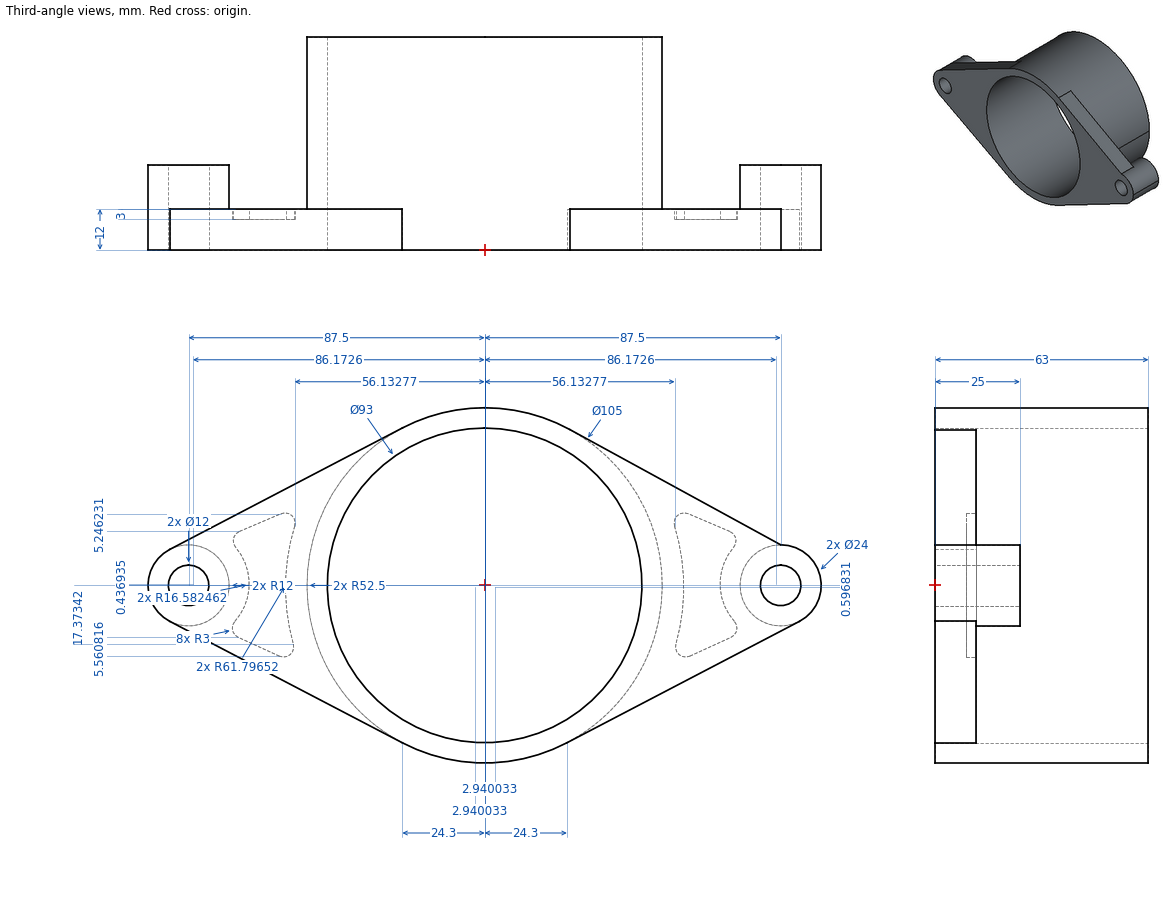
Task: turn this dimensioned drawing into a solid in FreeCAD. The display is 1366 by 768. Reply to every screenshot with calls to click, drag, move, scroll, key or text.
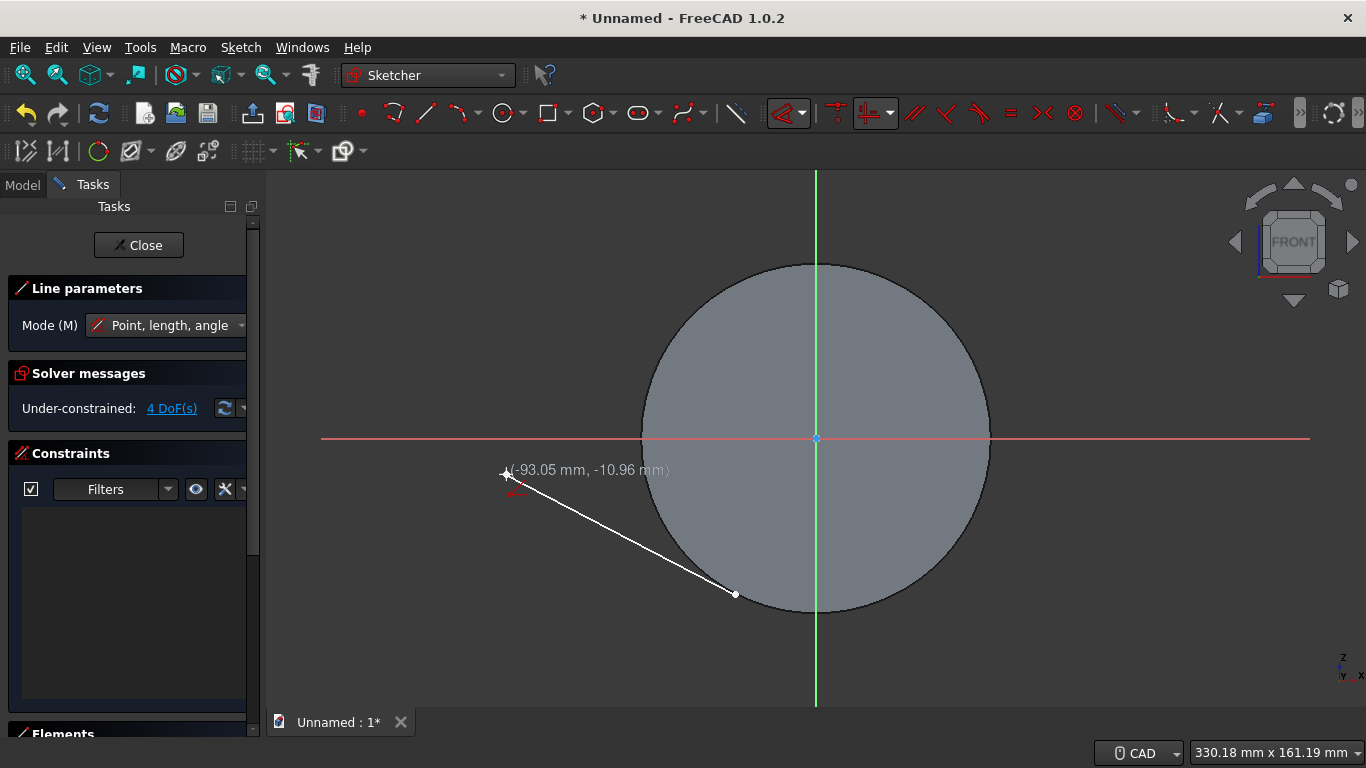
click(506, 403)
click(735, 283)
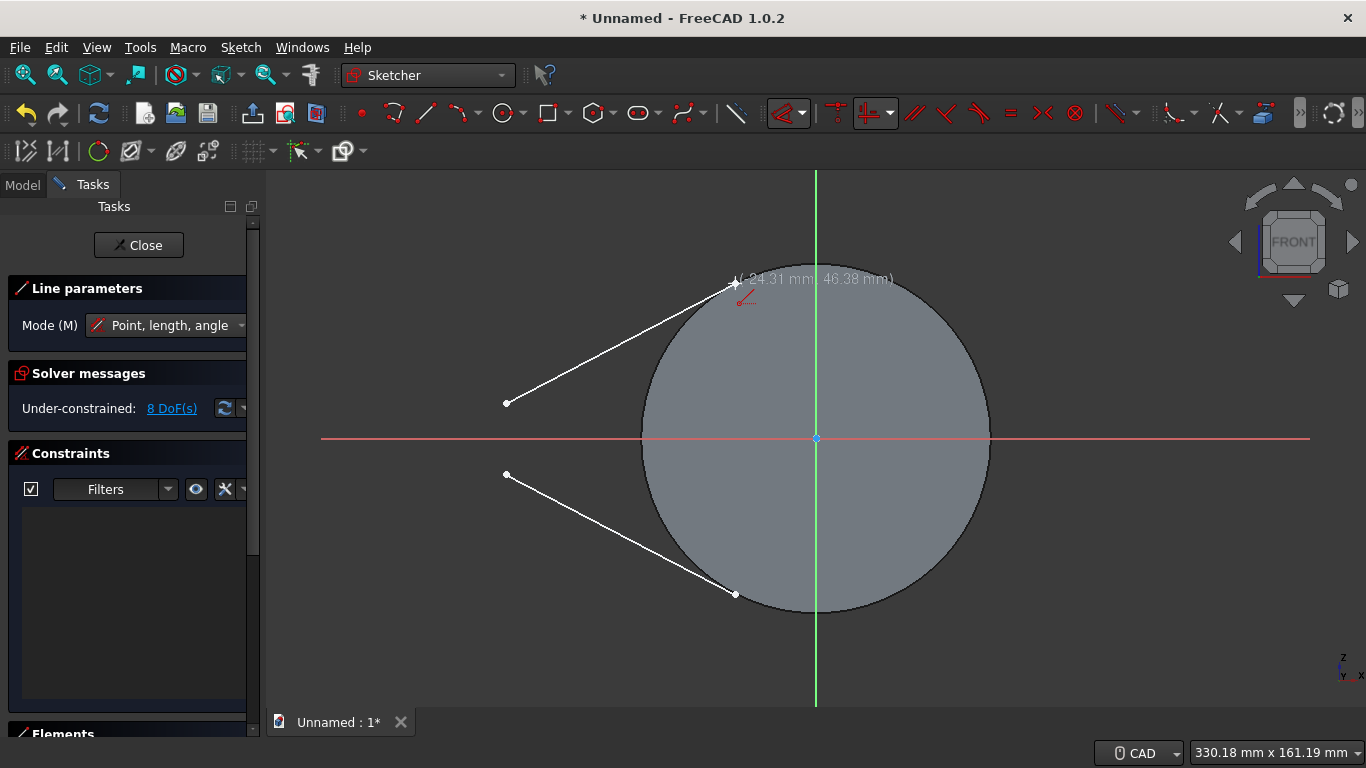
key(g)
key(3)
key(a)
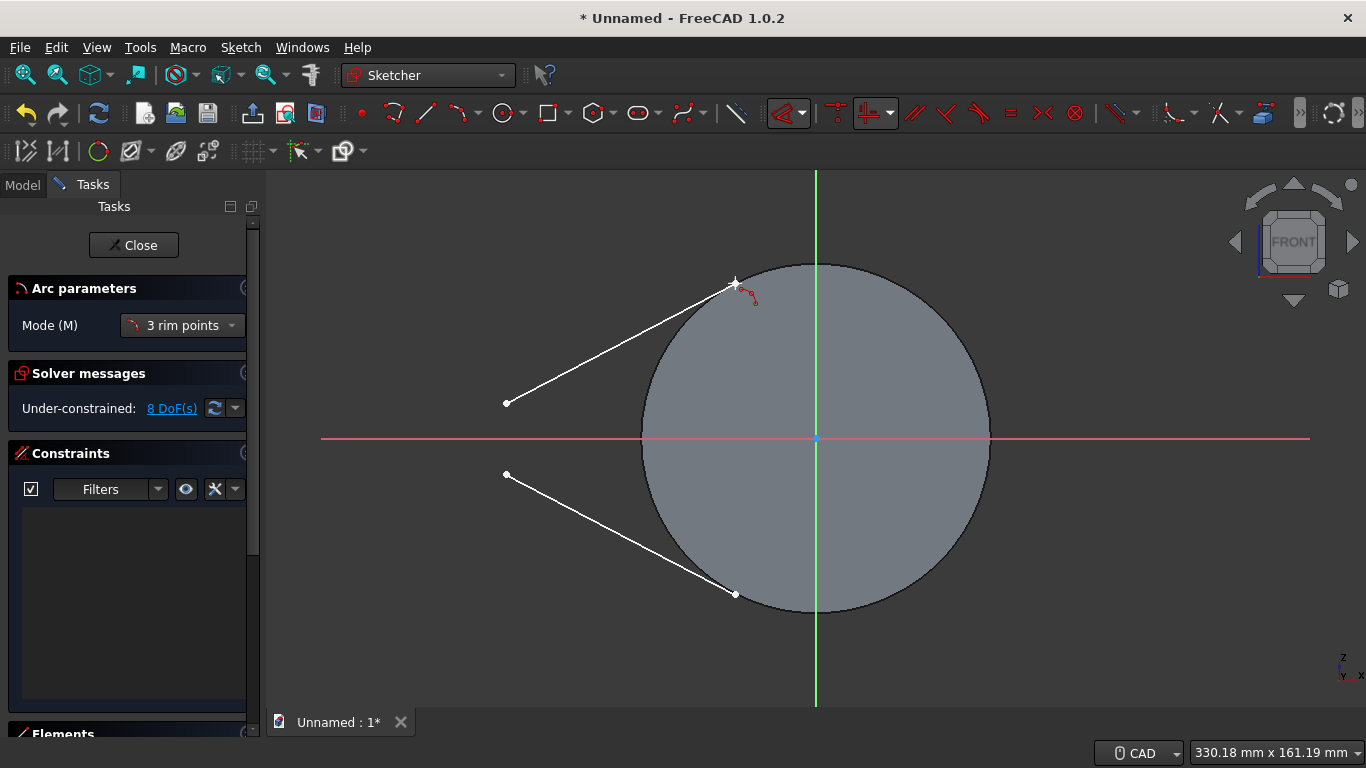
click(506, 475)
click(506, 404)
click(561, 454)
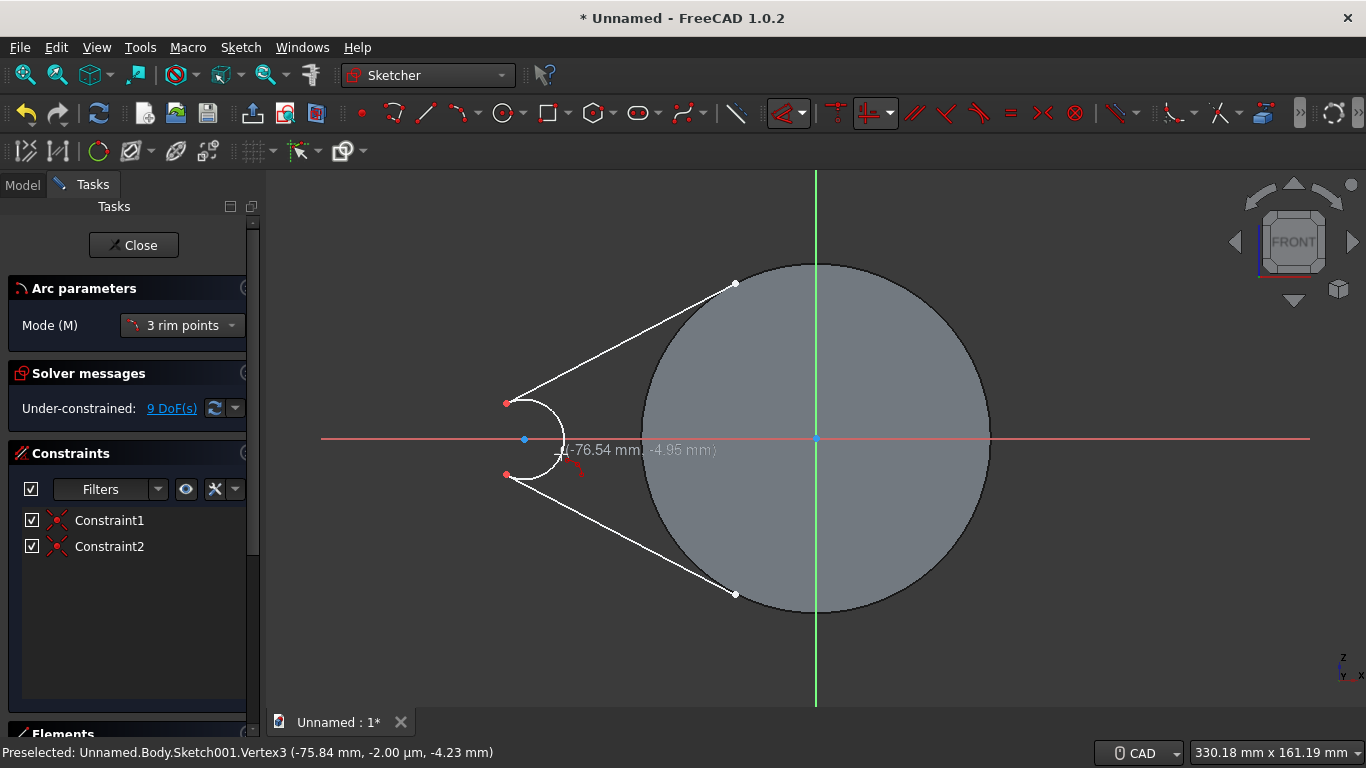
click(735, 284)
click(735, 595)
click(645, 401)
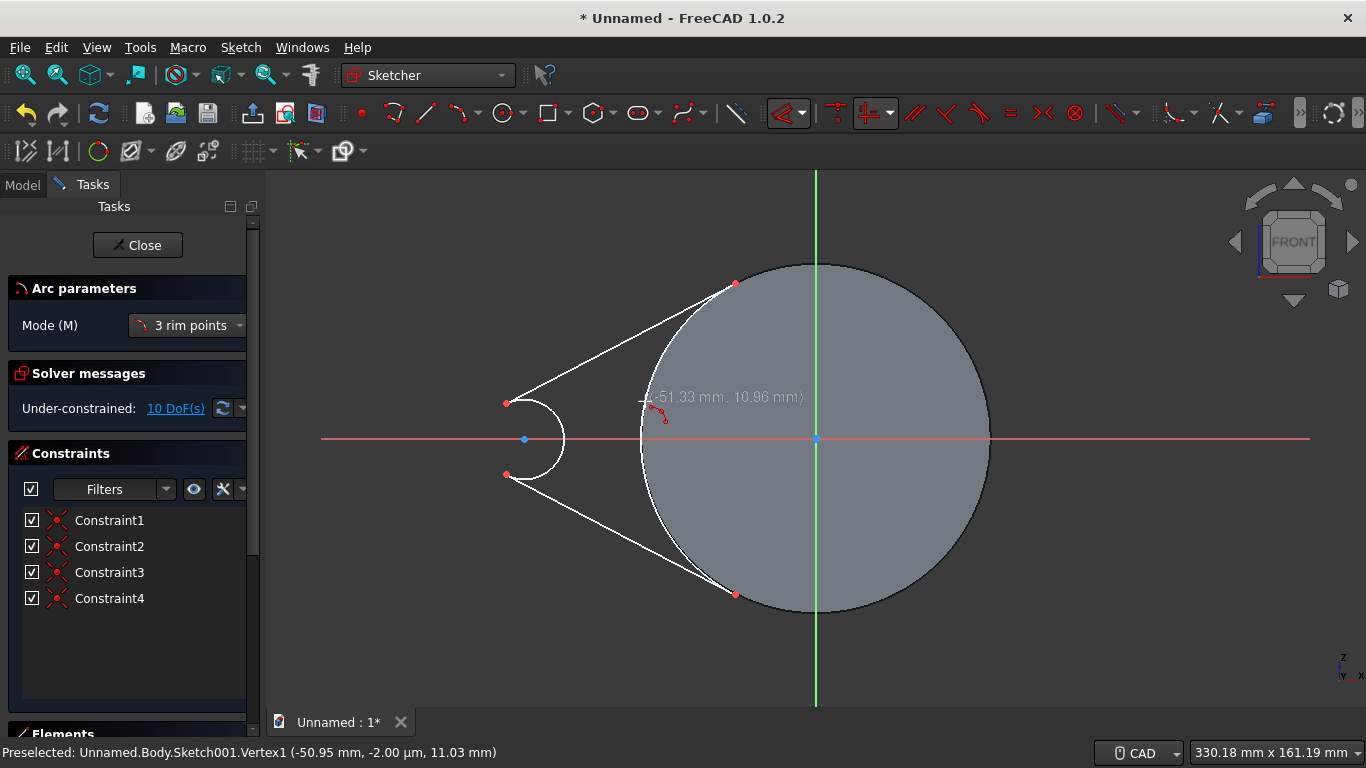
key(g)
key(l)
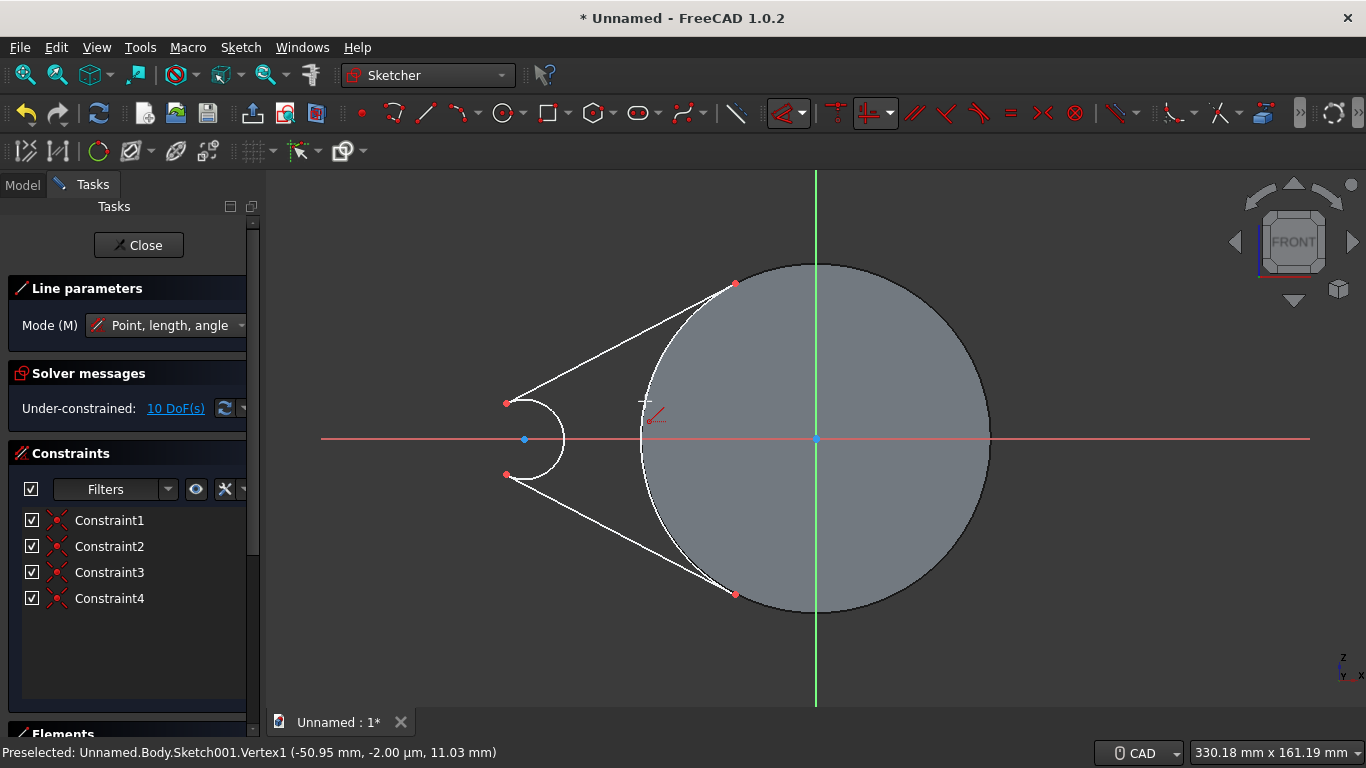
click(1126, 474)
click(897, 594)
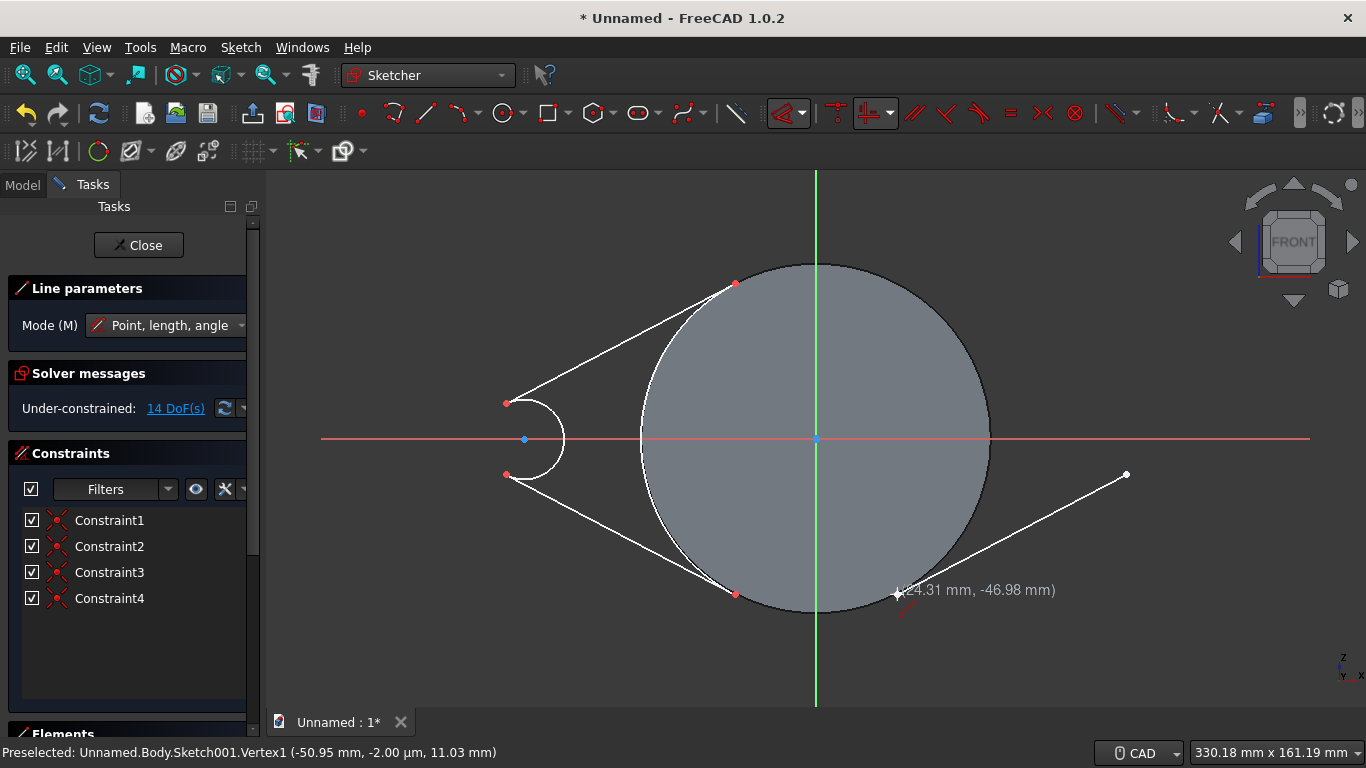
click(900, 285)
click(1108, 399)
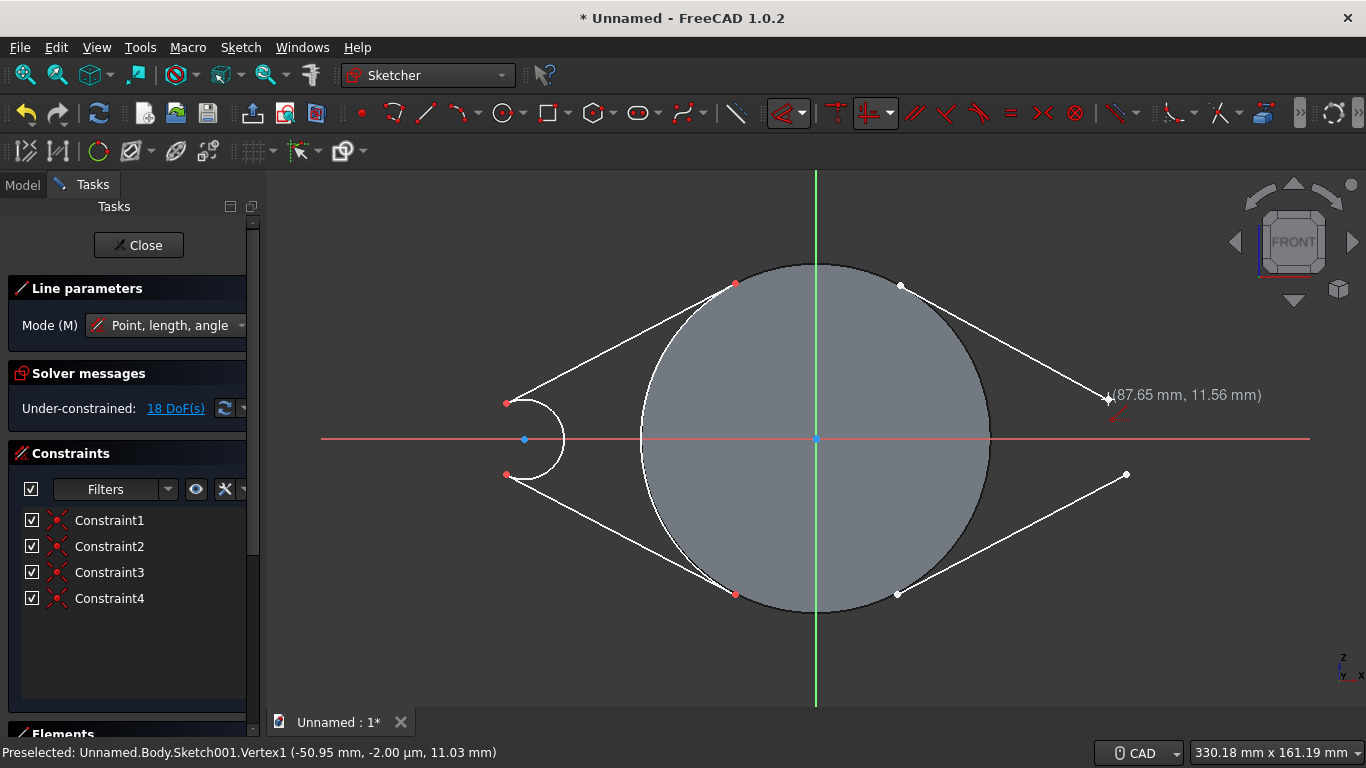
key(g)
key(3)
key(a)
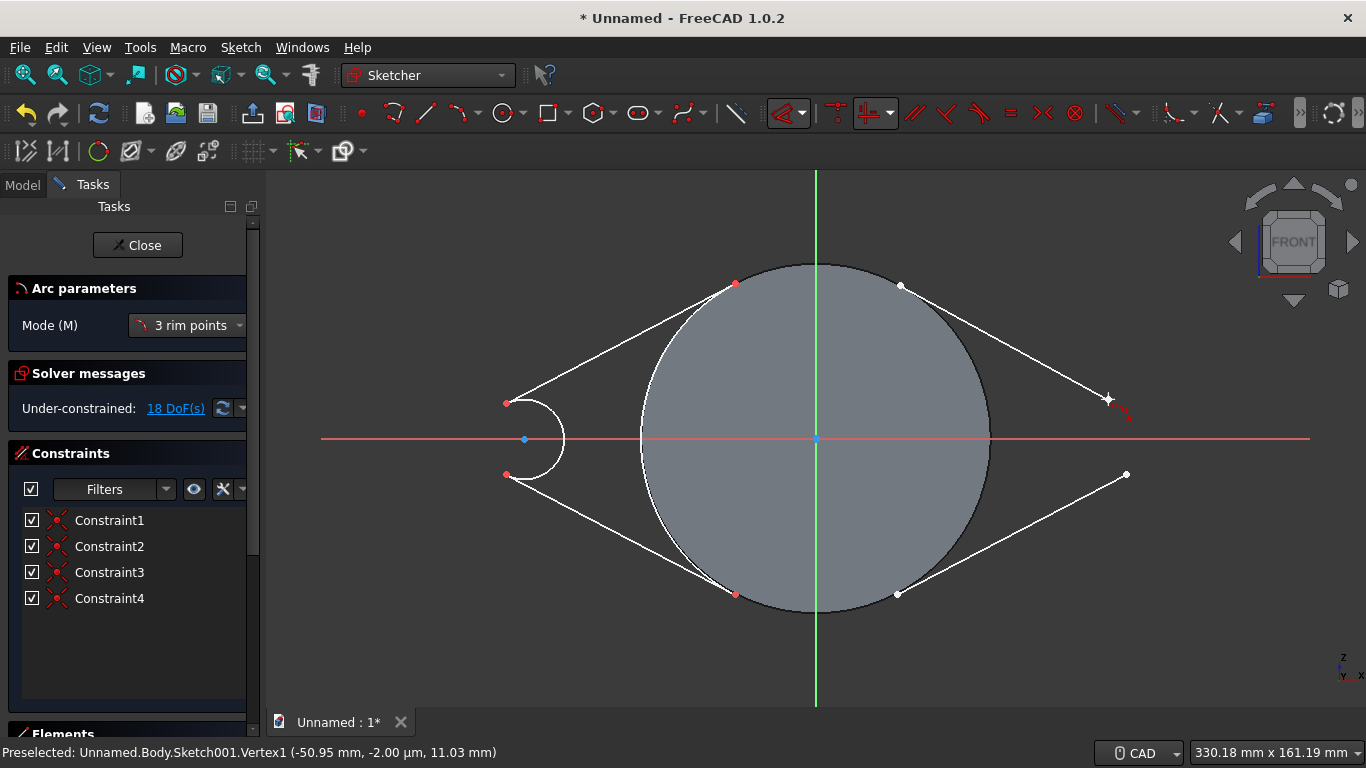
click(897, 595)
click(900, 286)
click(986, 478)